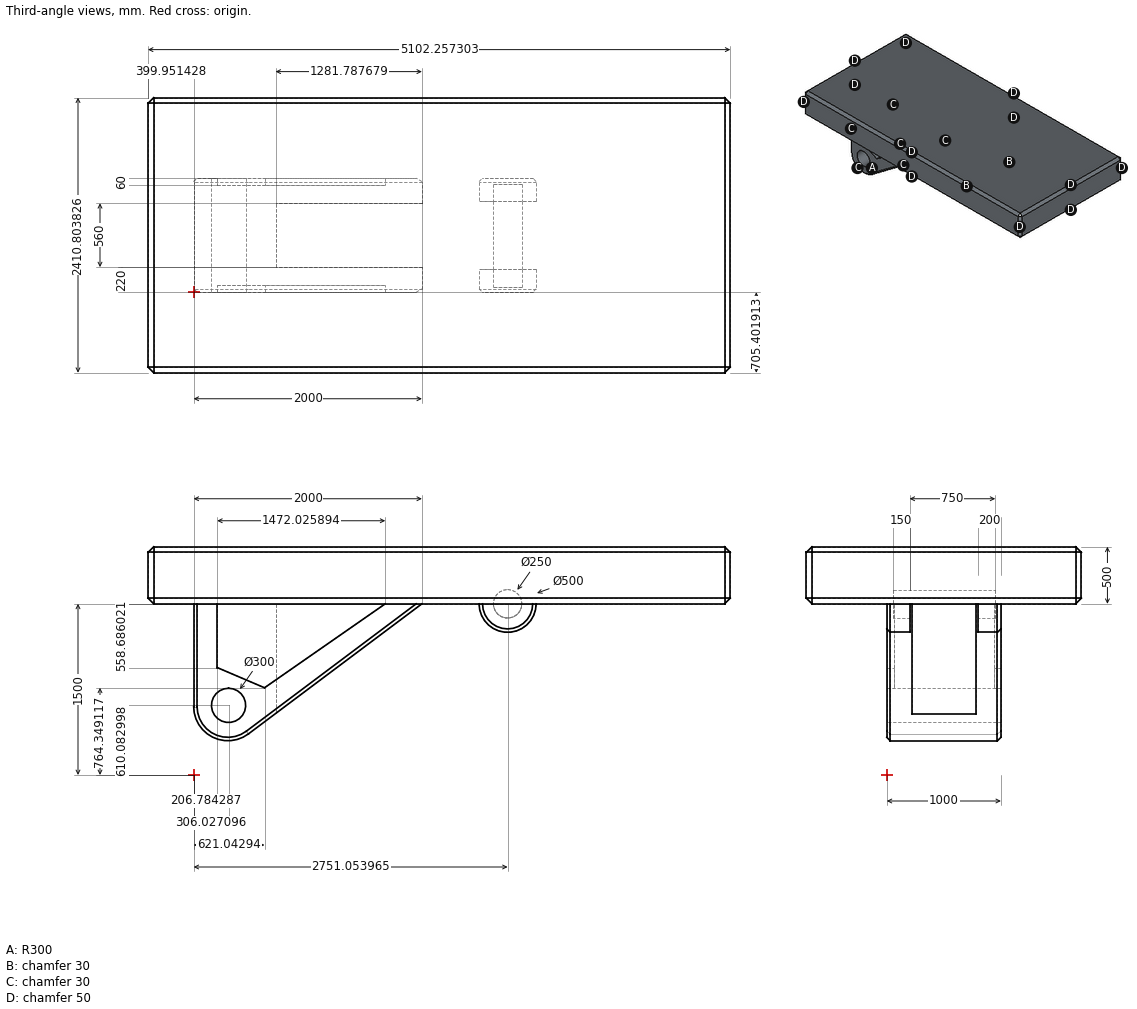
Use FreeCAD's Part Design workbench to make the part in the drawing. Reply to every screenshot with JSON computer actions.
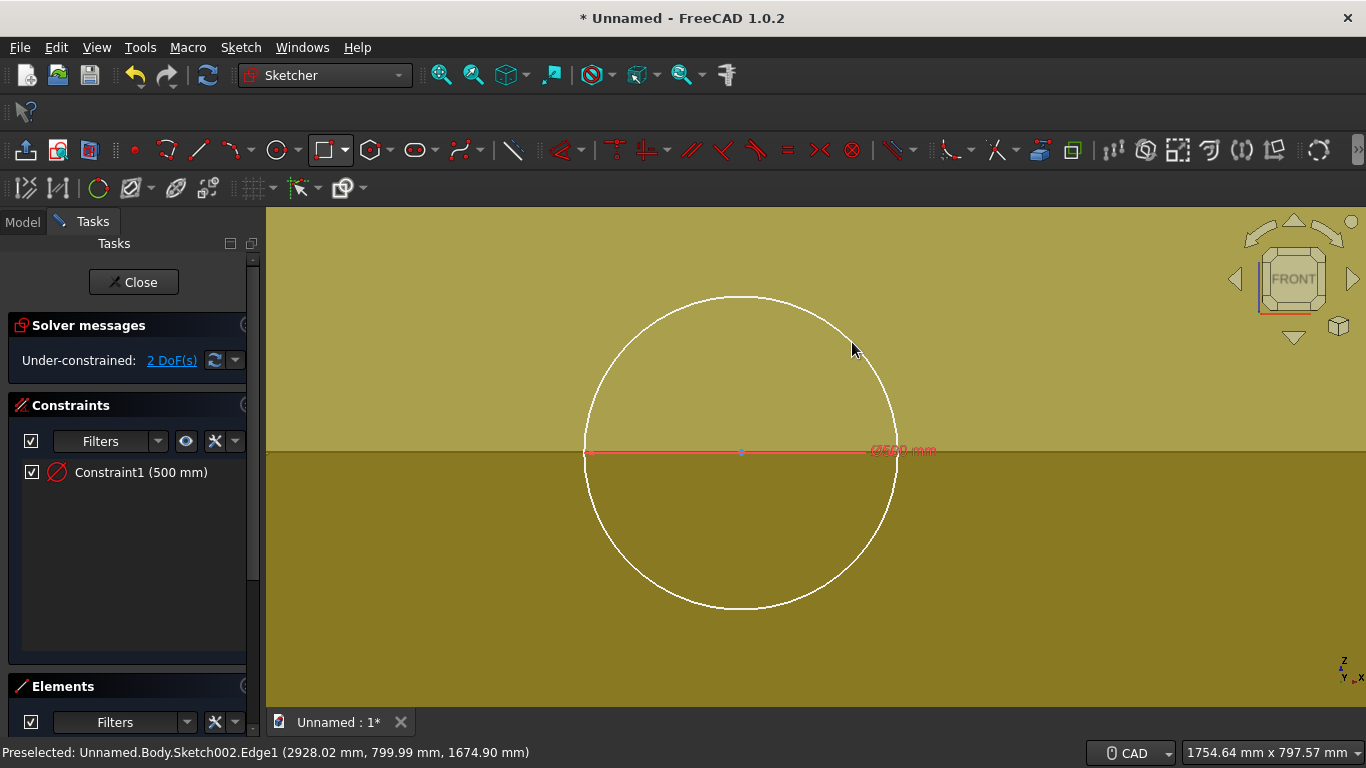
{"action": "left_click", "coordinate": [560, 150]}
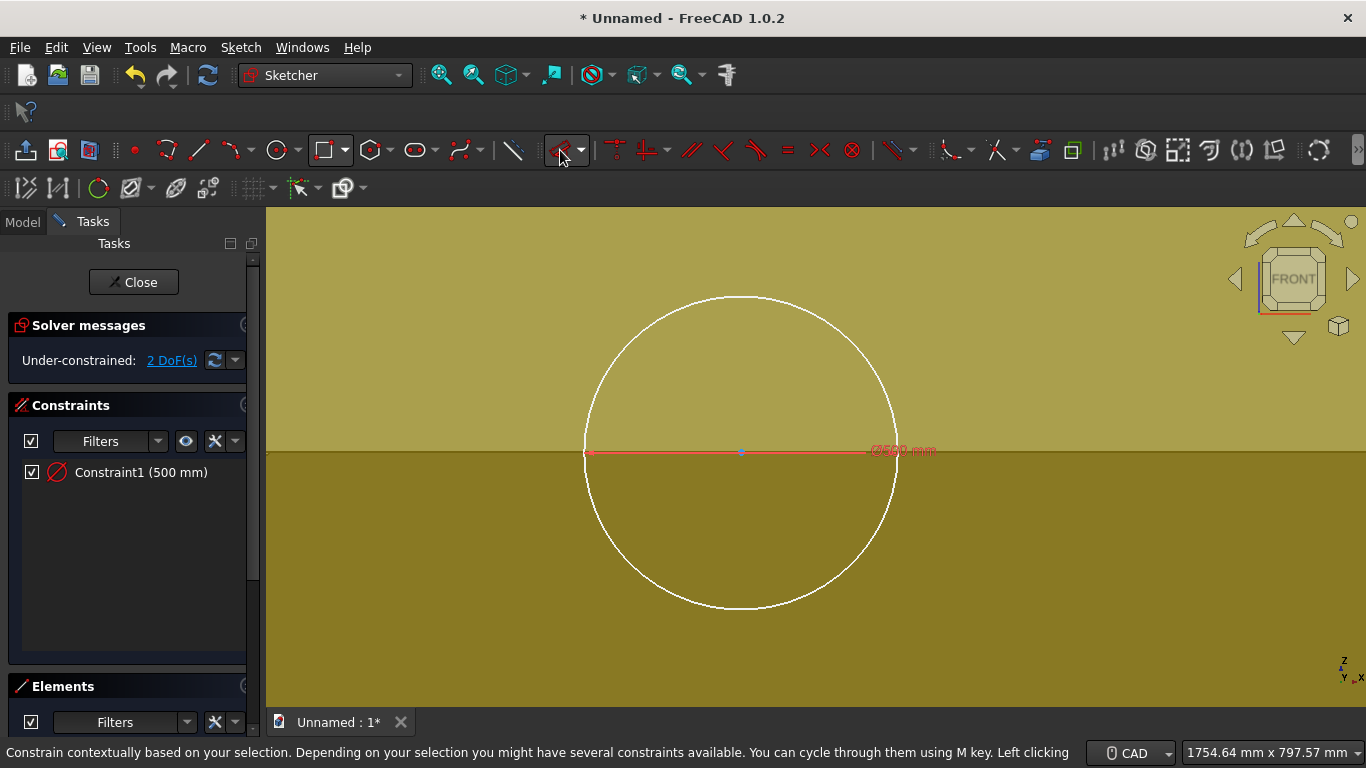
{"action": "left_click", "coordinate": [741, 453]}
{"action": "left_click", "coordinate": [775, 566]}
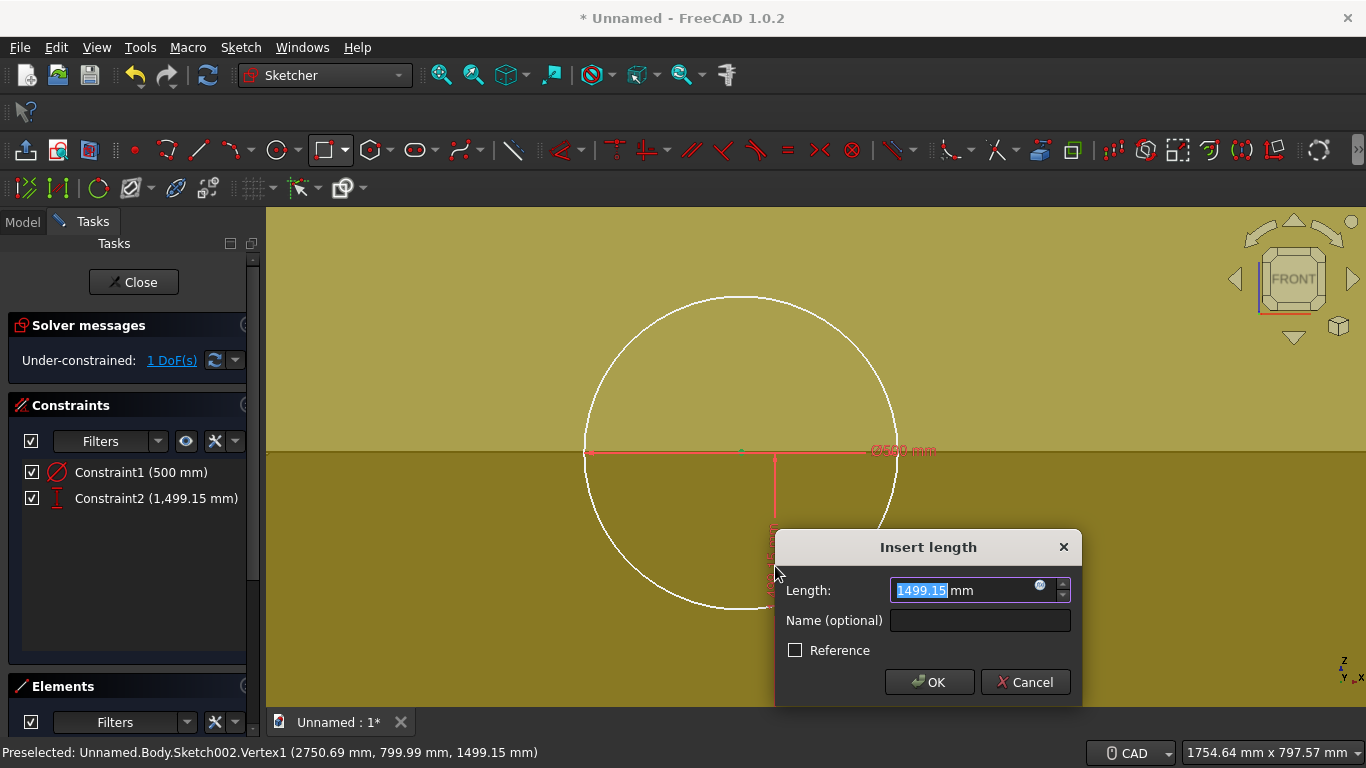
{"action": "type", "text": "1500"}
{"action": "key", "text": "Return"}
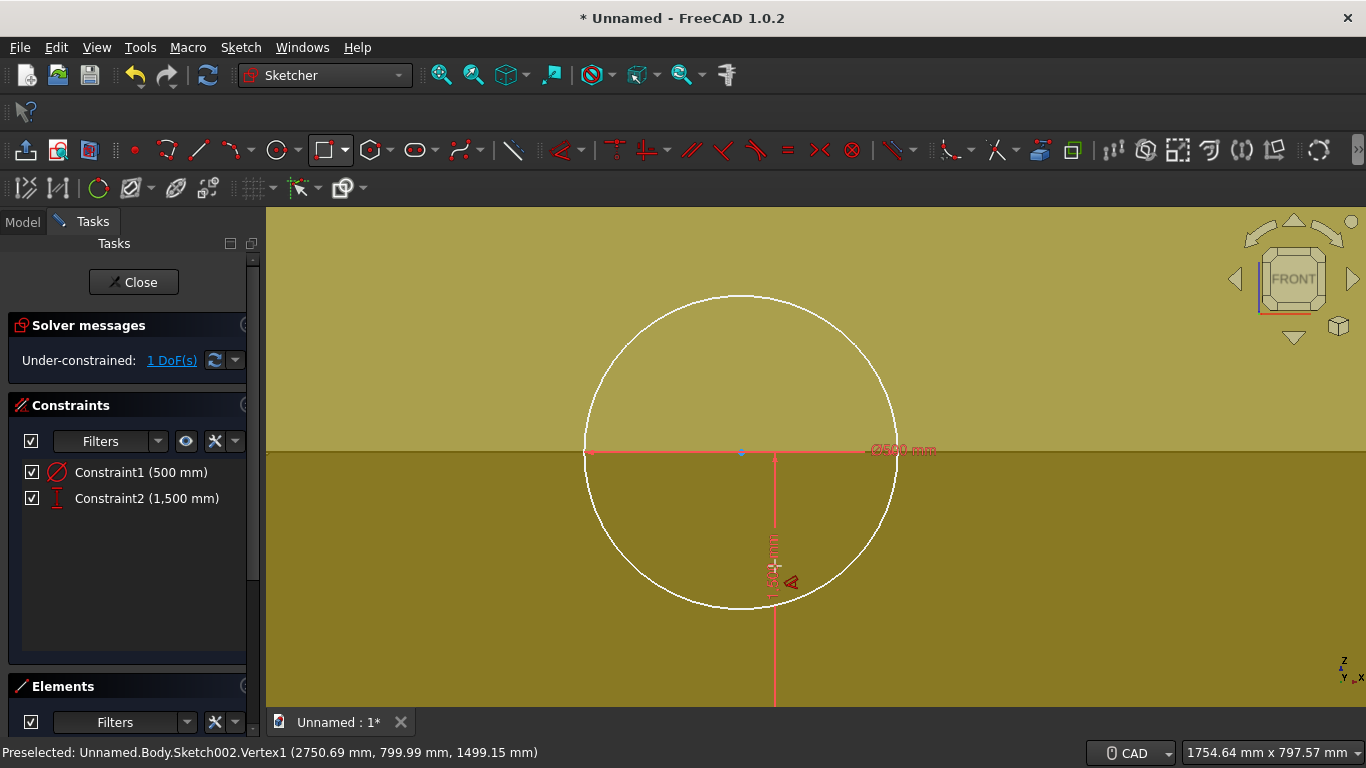
{"action": "left_click", "coordinate": [741, 452]}
{"action": "left_click", "coordinate": [518, 418]}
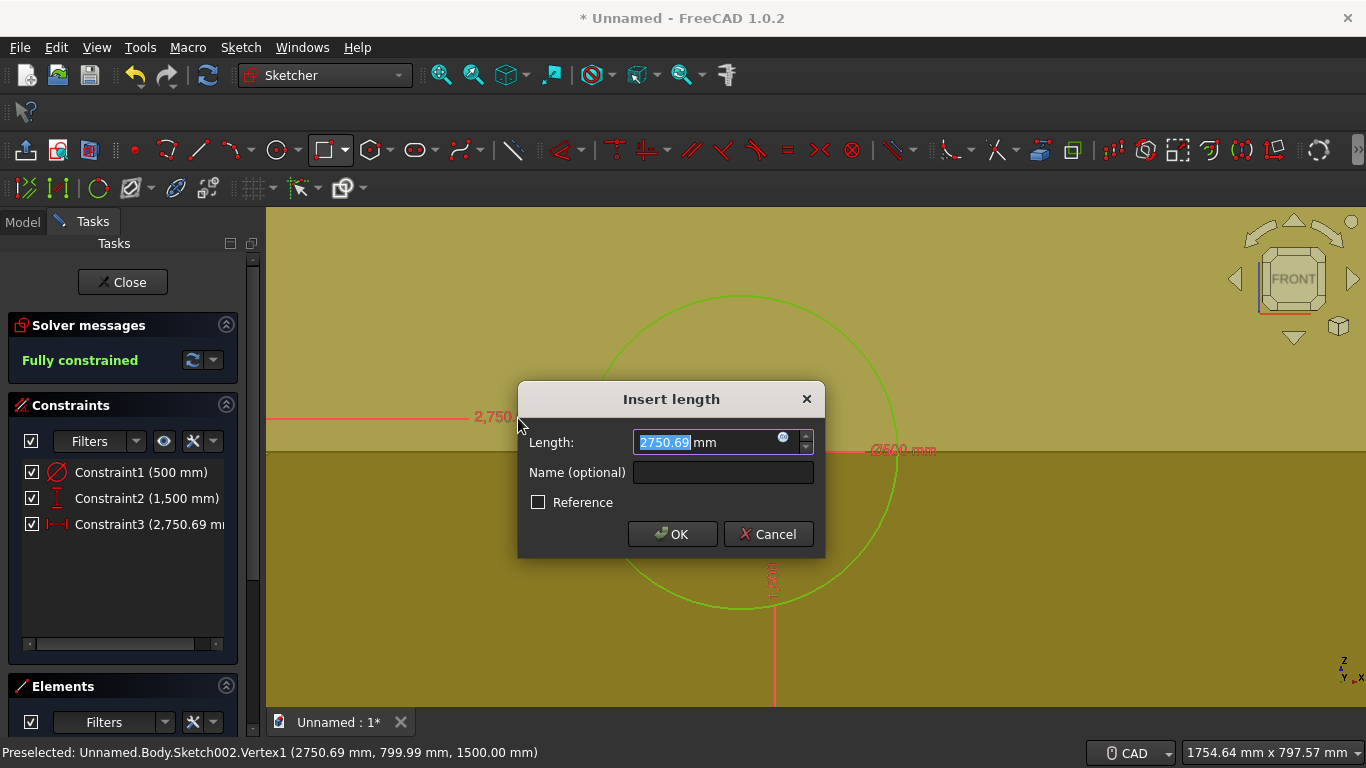
{"action": "type", "text": "2751.053965"}
{"action": "key", "text": "Return"}
{"action": "key", "text": "Escape"}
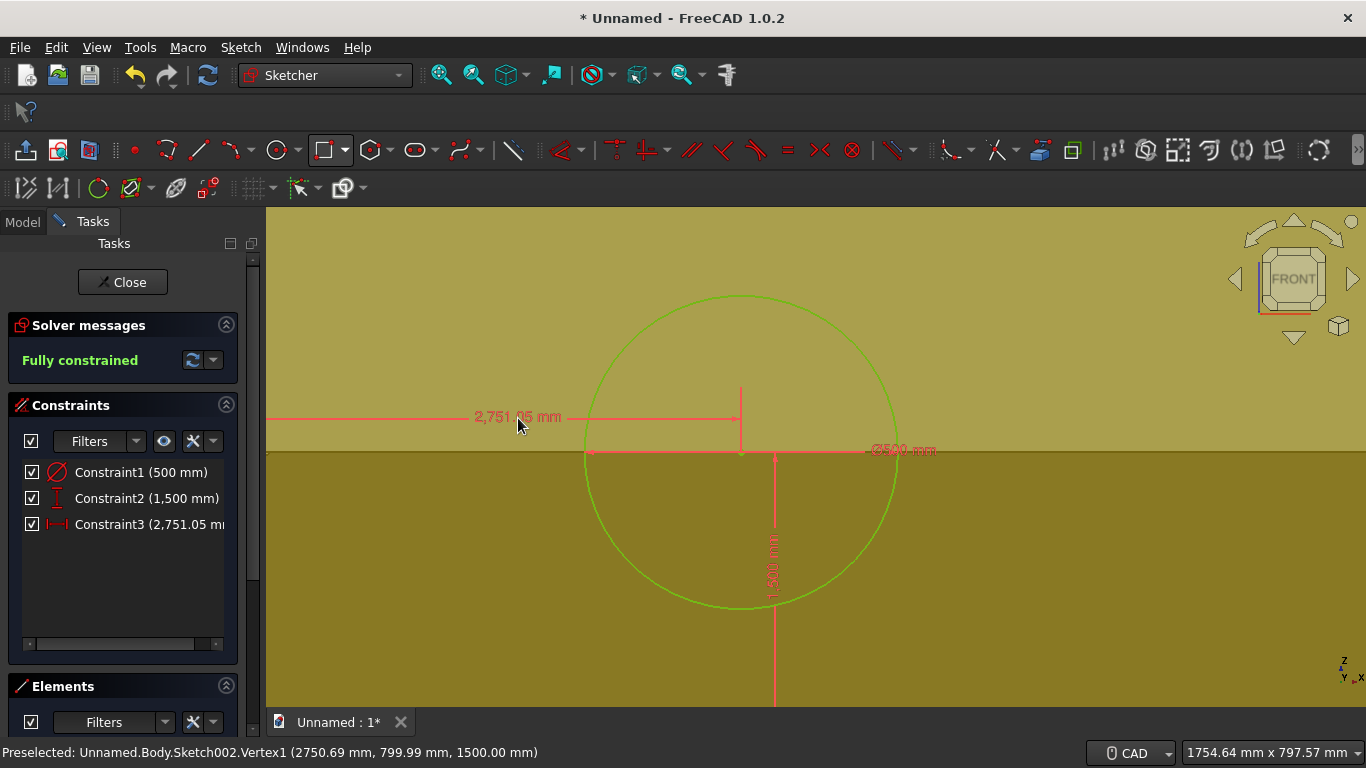
{"action": "left_click", "coordinate": [123, 282]}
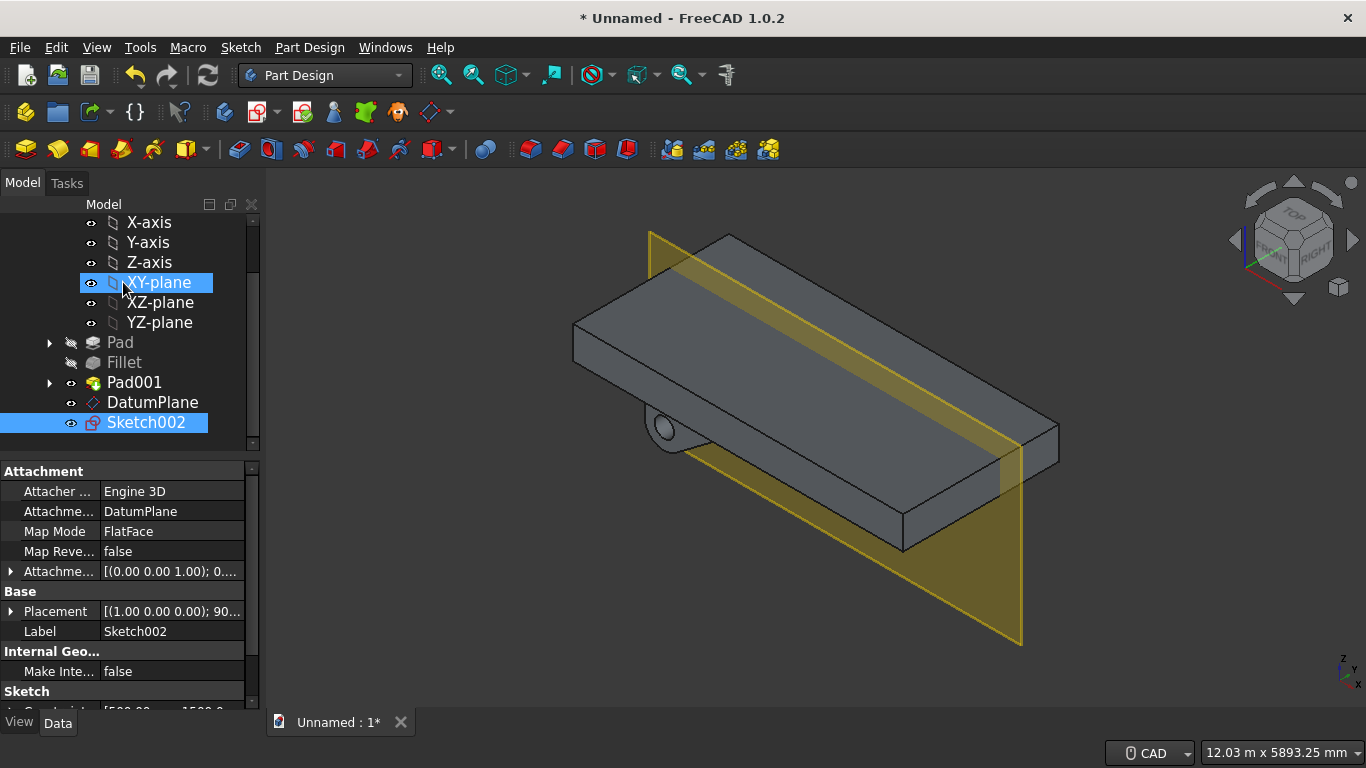
{"action": "left_click", "coordinate": [26, 150]}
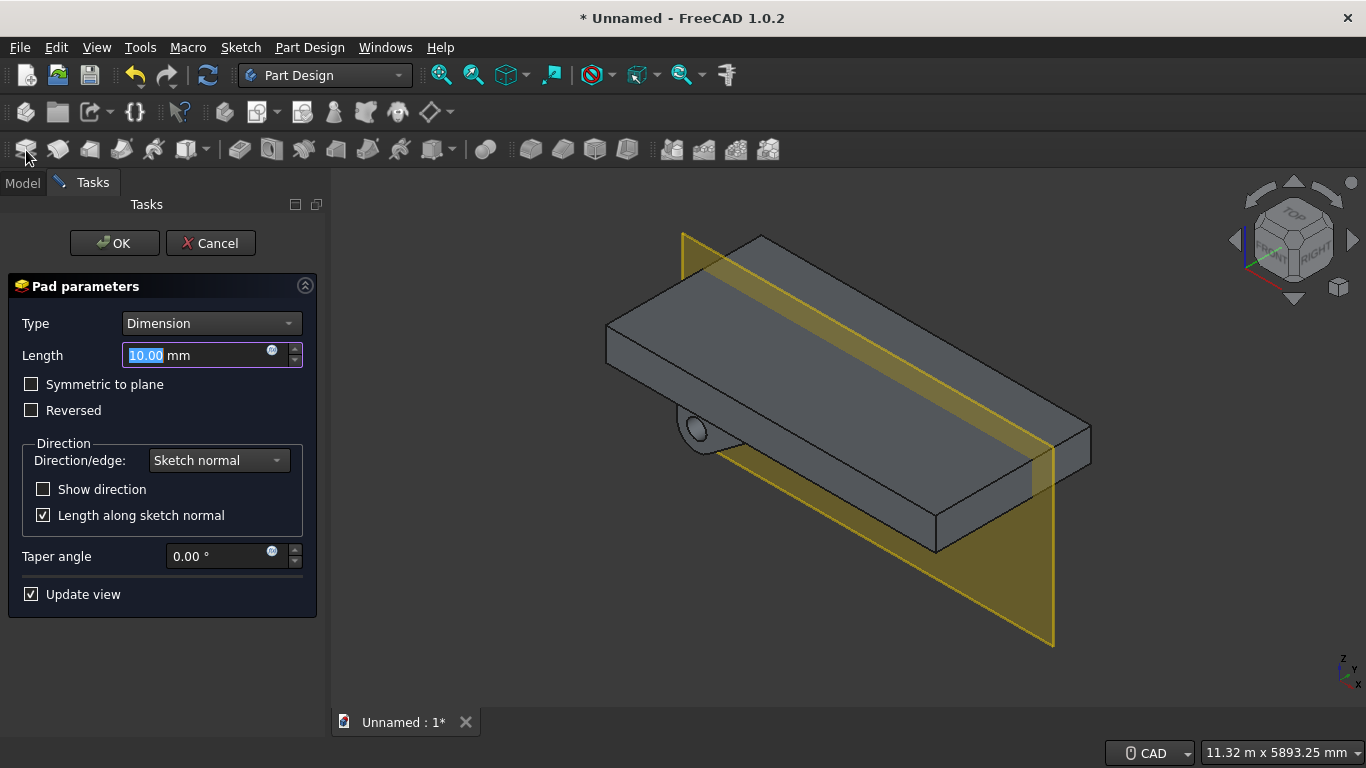
{"action": "type", "text": "200"}
{"action": "key", "text": "Tab"}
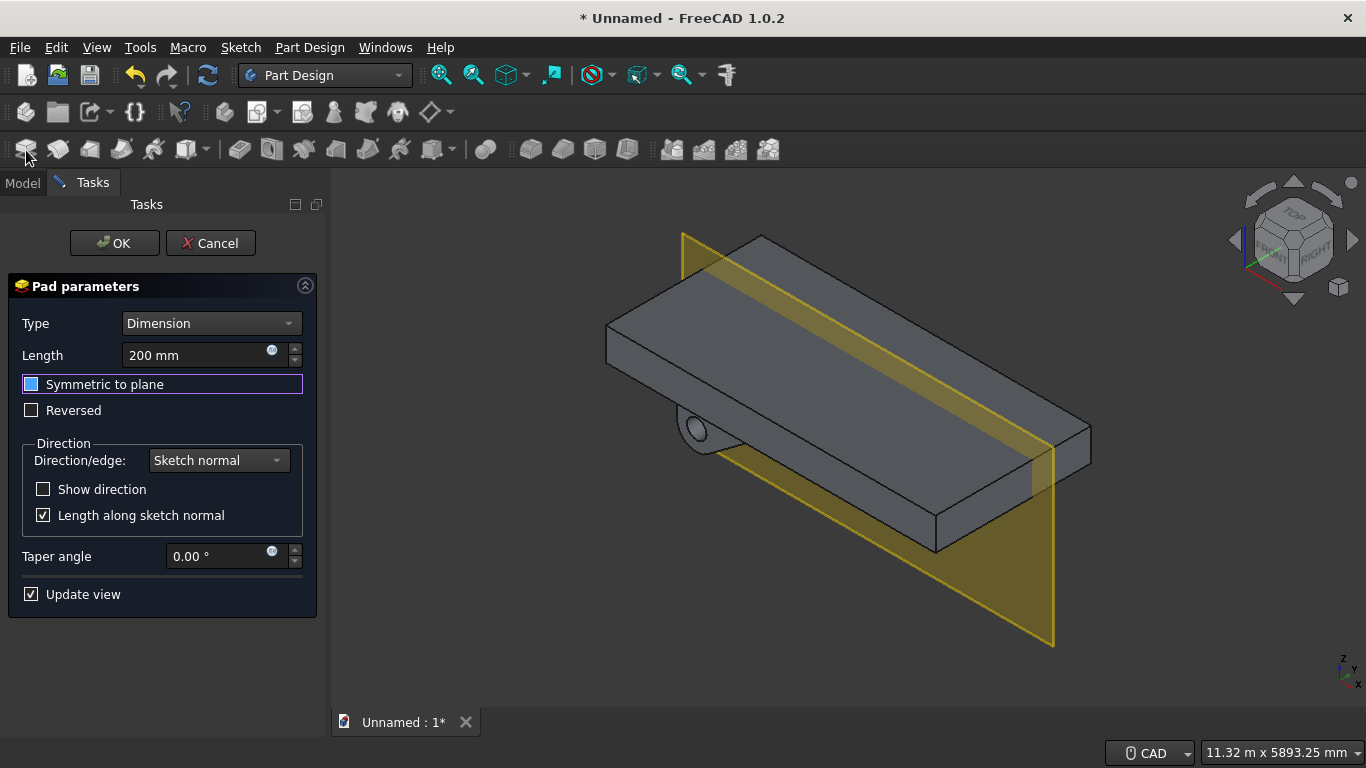
{"action": "left_click", "coordinate": [30, 410]}